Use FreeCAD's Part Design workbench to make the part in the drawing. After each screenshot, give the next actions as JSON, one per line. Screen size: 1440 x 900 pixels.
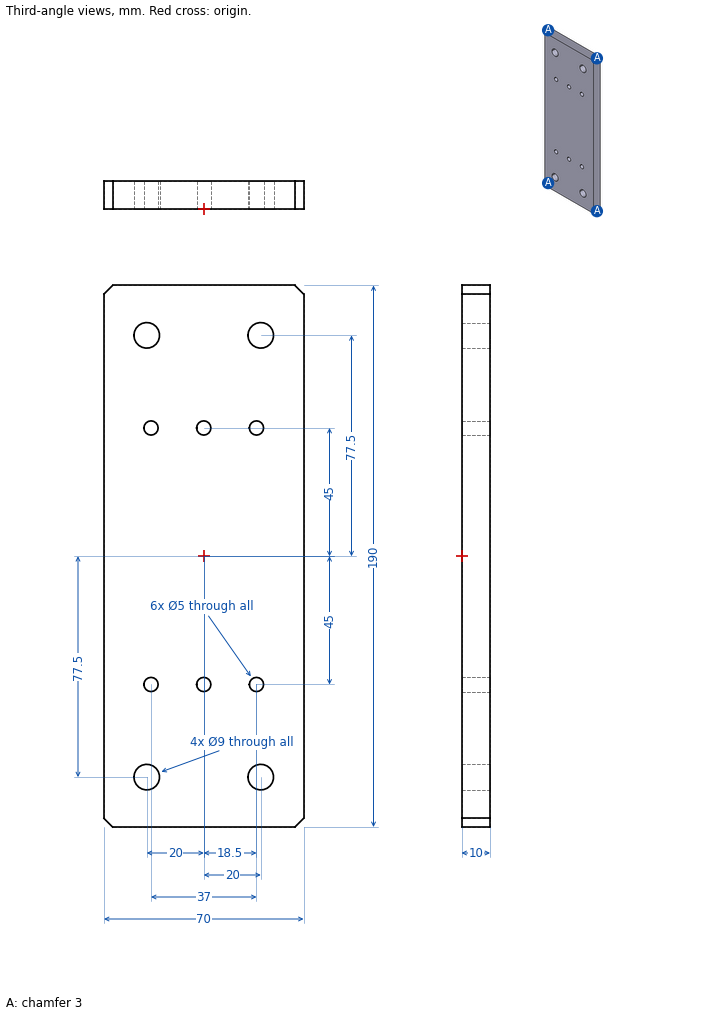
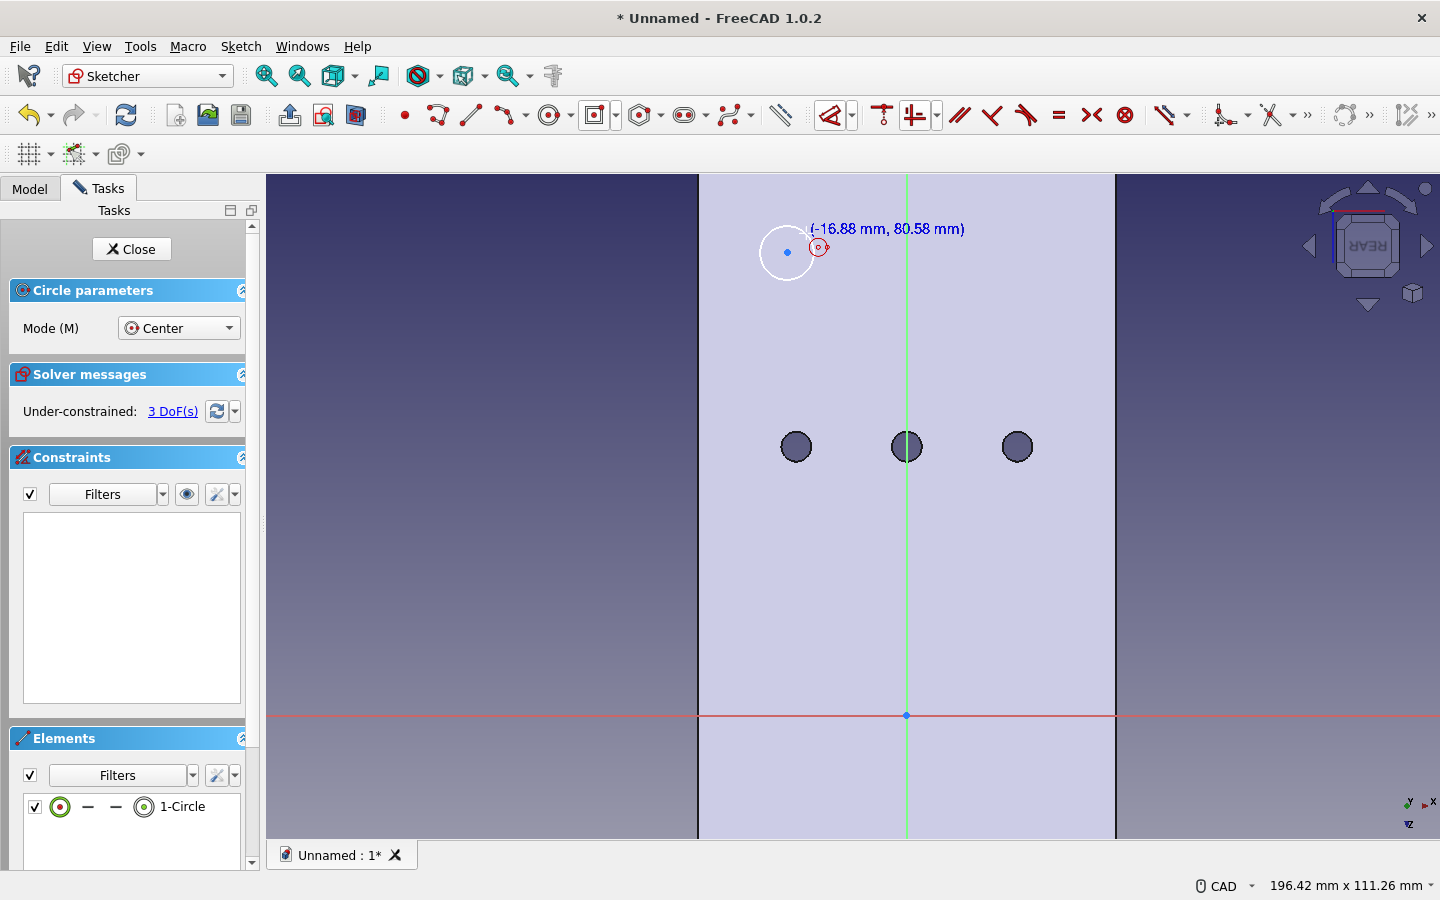
{"action": "left_click", "coordinate": [1026, 252]}
{"action": "left_click", "coordinate": [1045, 233]}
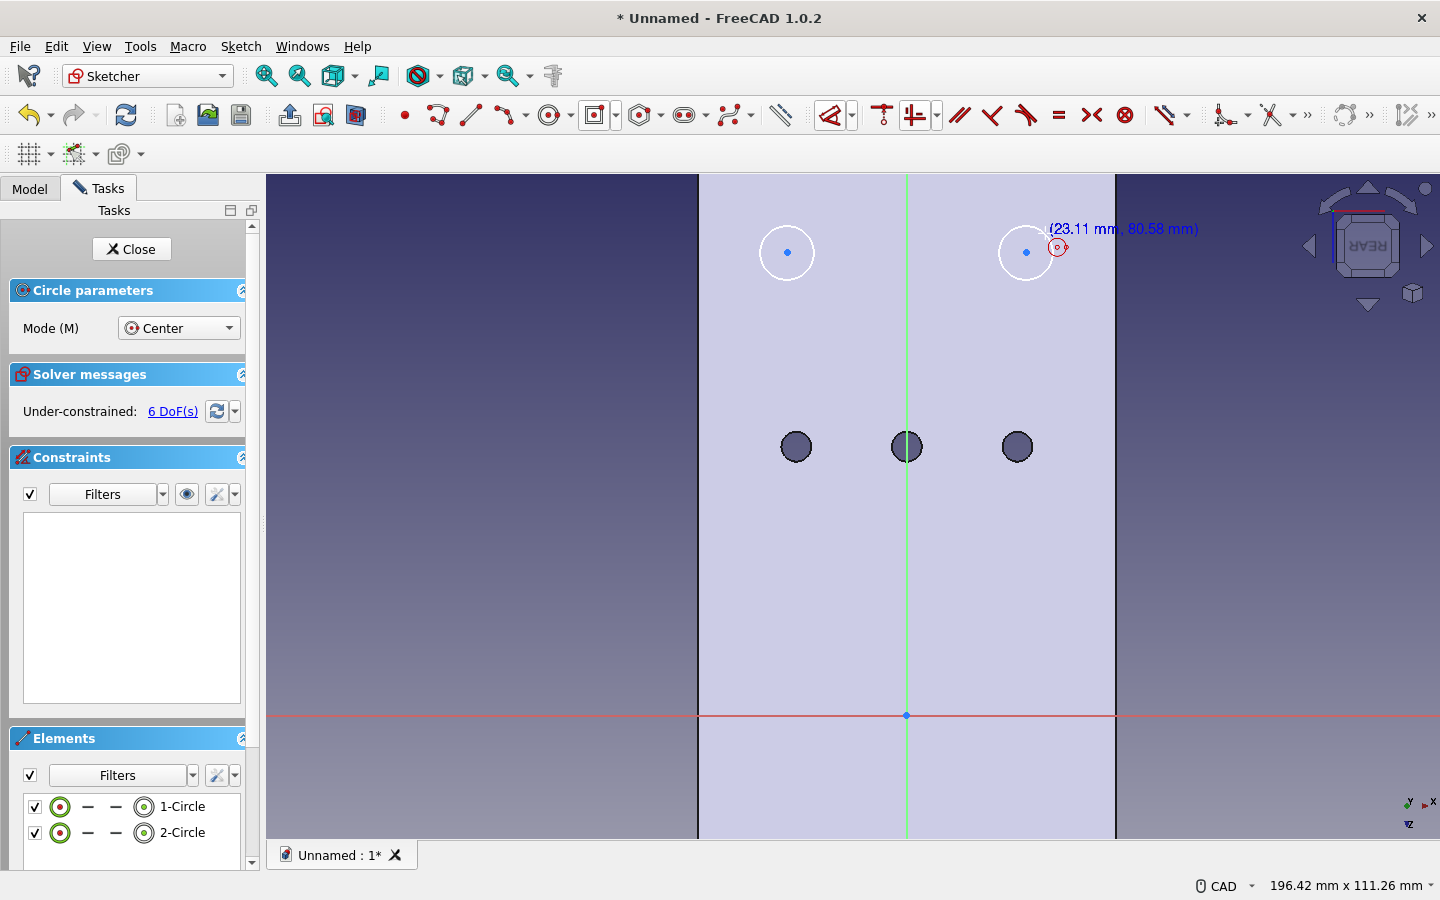
{"action": "scroll", "coordinate": [685, 336], "scroll_direction": "down", "scroll_amount": 4}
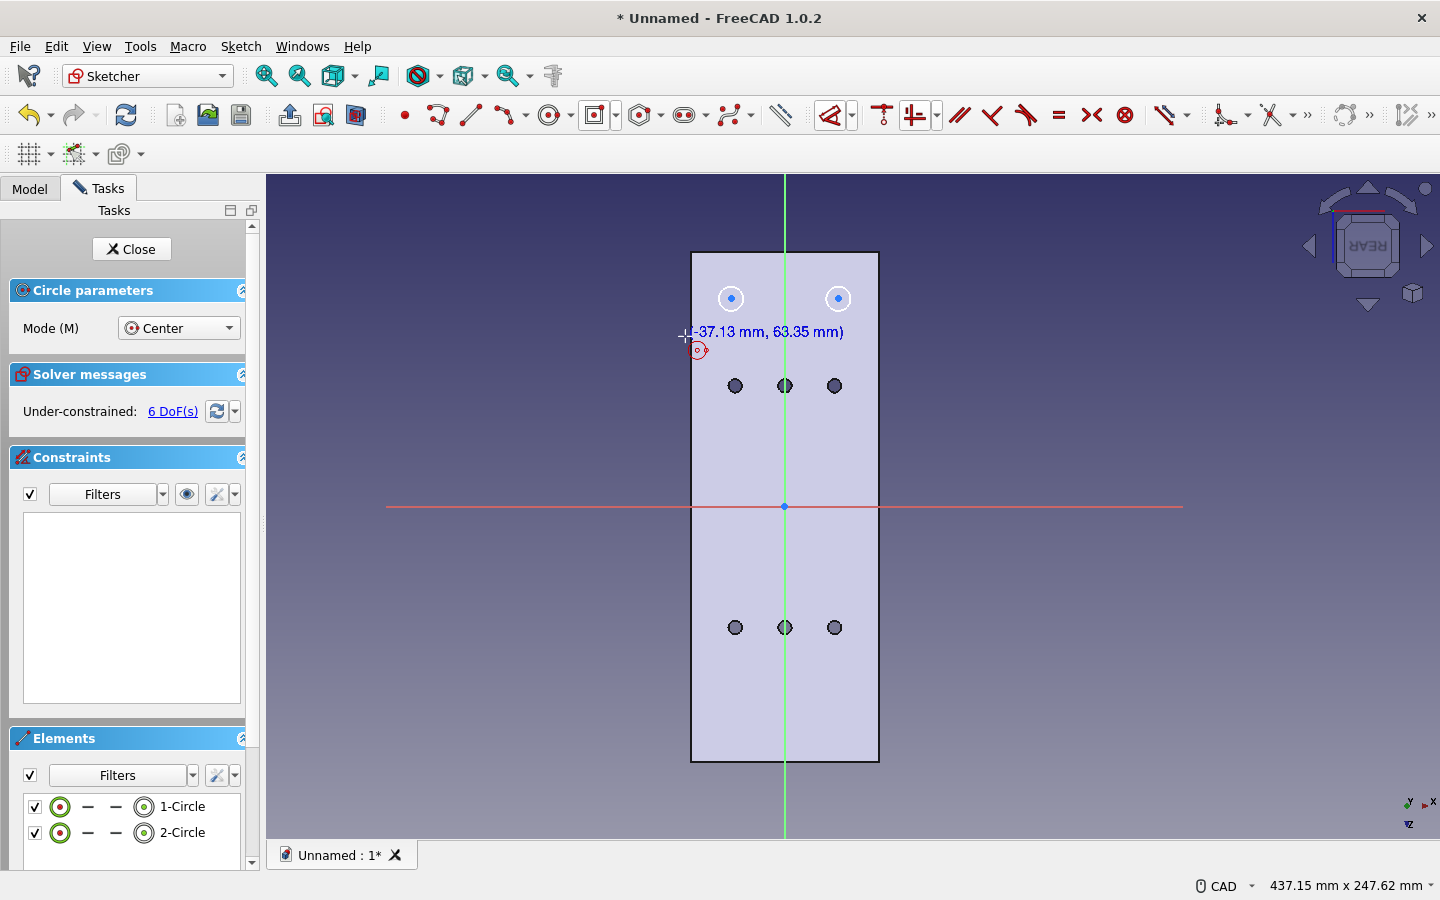
{"action": "scroll", "coordinate": [839, 715], "scroll_direction": "up", "scroll_amount": 4}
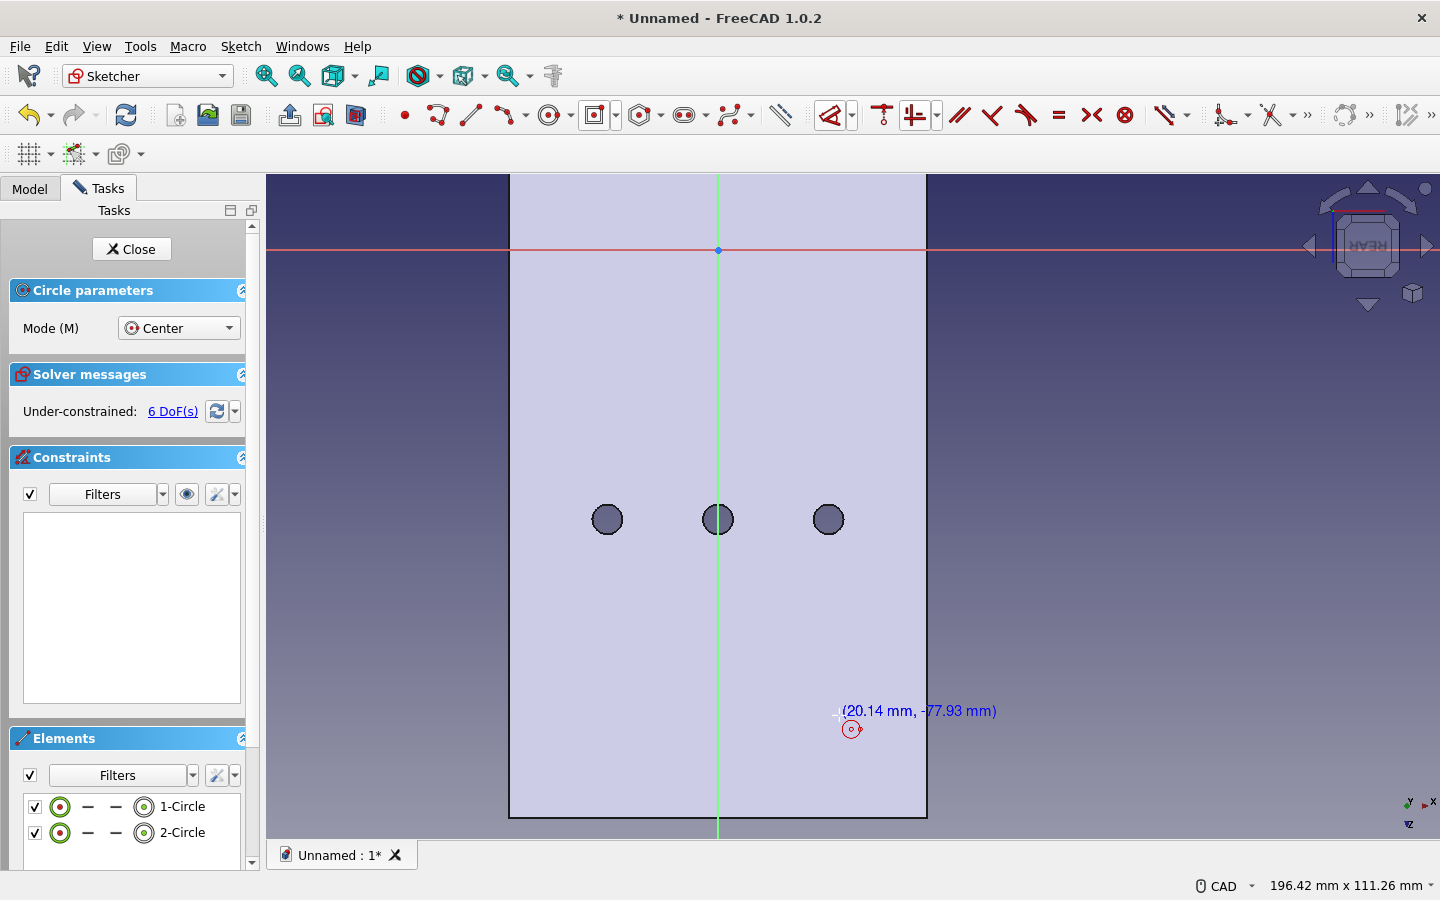
{"action": "left_click", "coordinate": [838, 714]}
{"action": "left_click", "coordinate": [857, 695]}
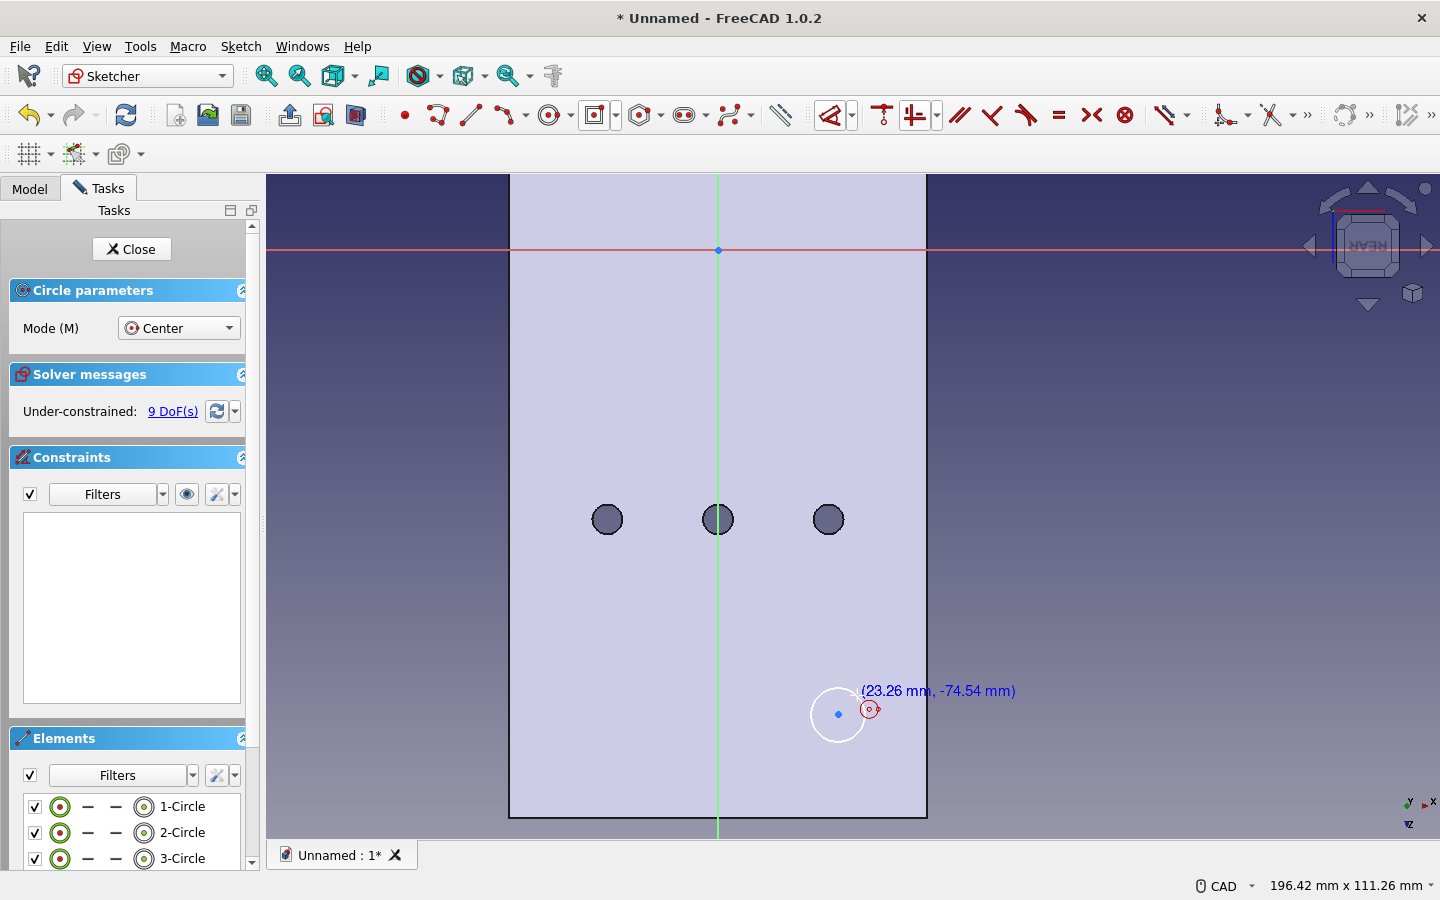
{"action": "left_click", "coordinate": [598, 714]}
{"action": "left_click", "coordinate": [617, 695]}
{"action": "key", "text": "Escape"}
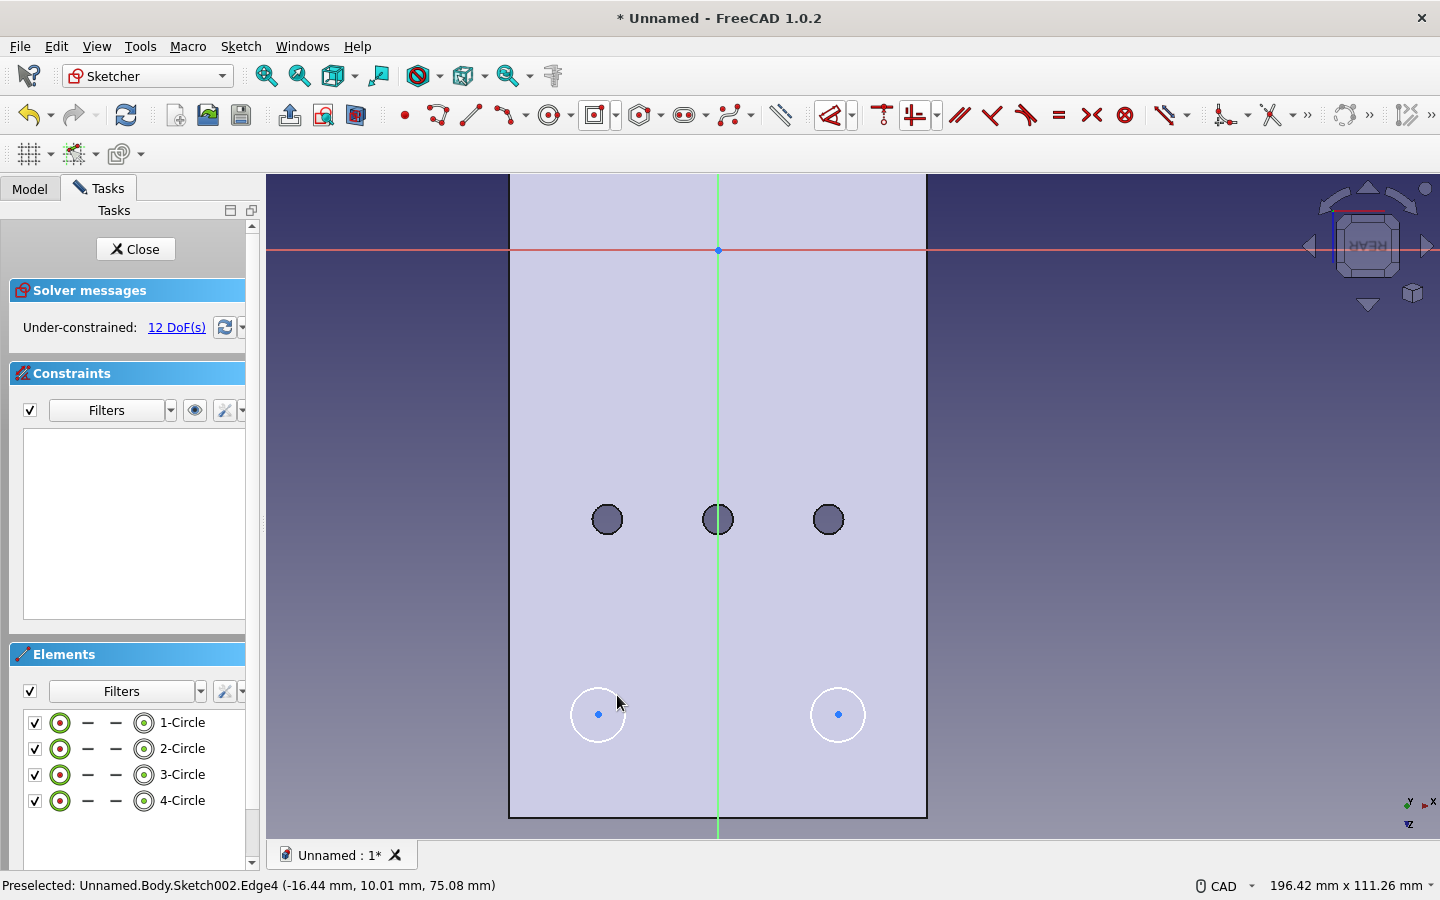
{"action": "scroll", "coordinate": [839, 715], "scroll_direction": "down", "scroll_amount": 4}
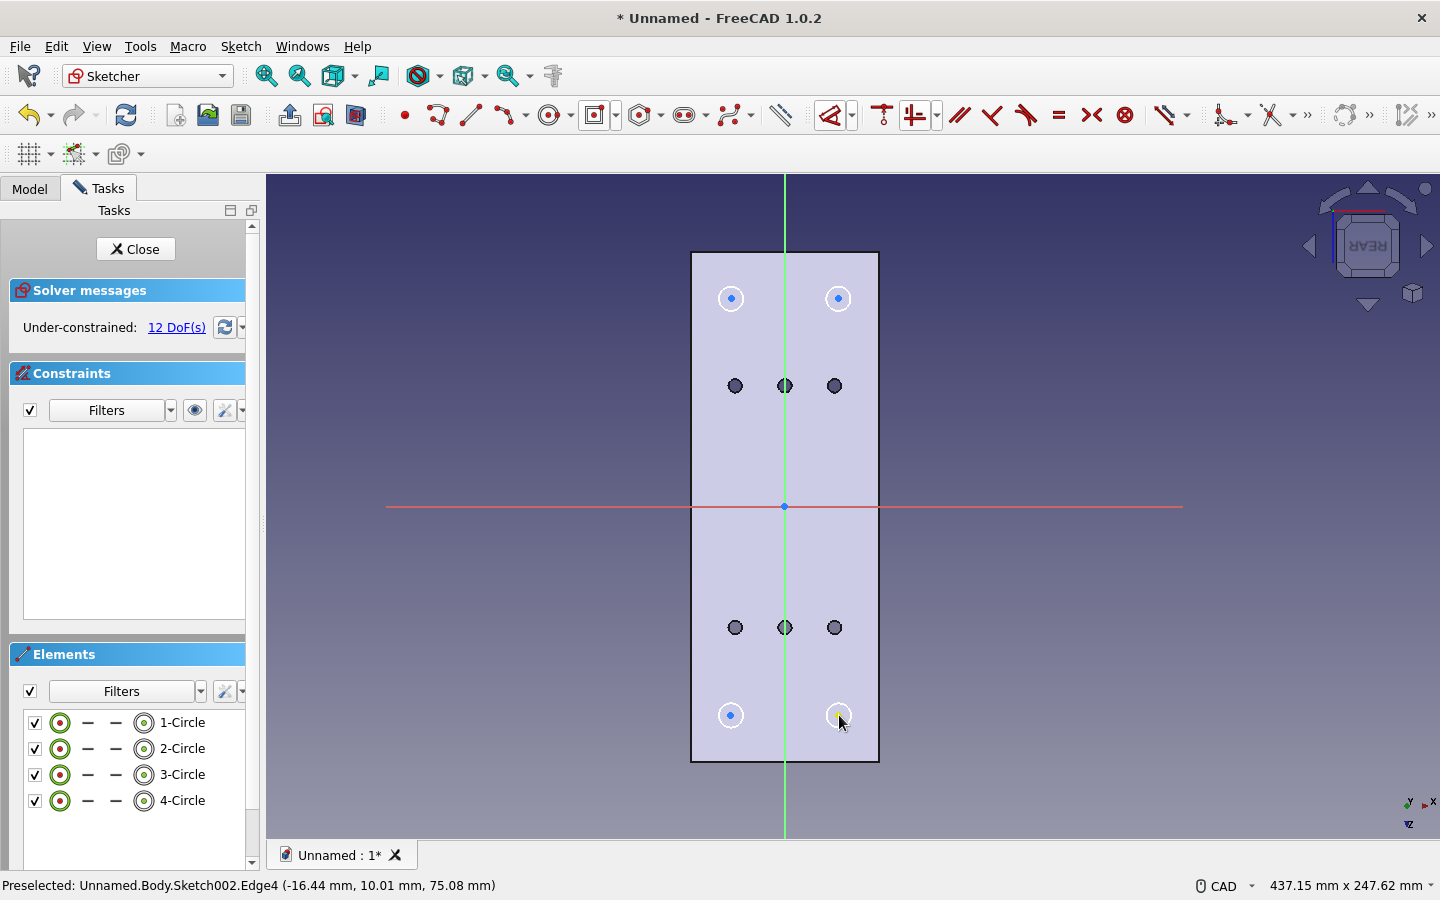
{"action": "left_click", "coordinate": [740, 290]}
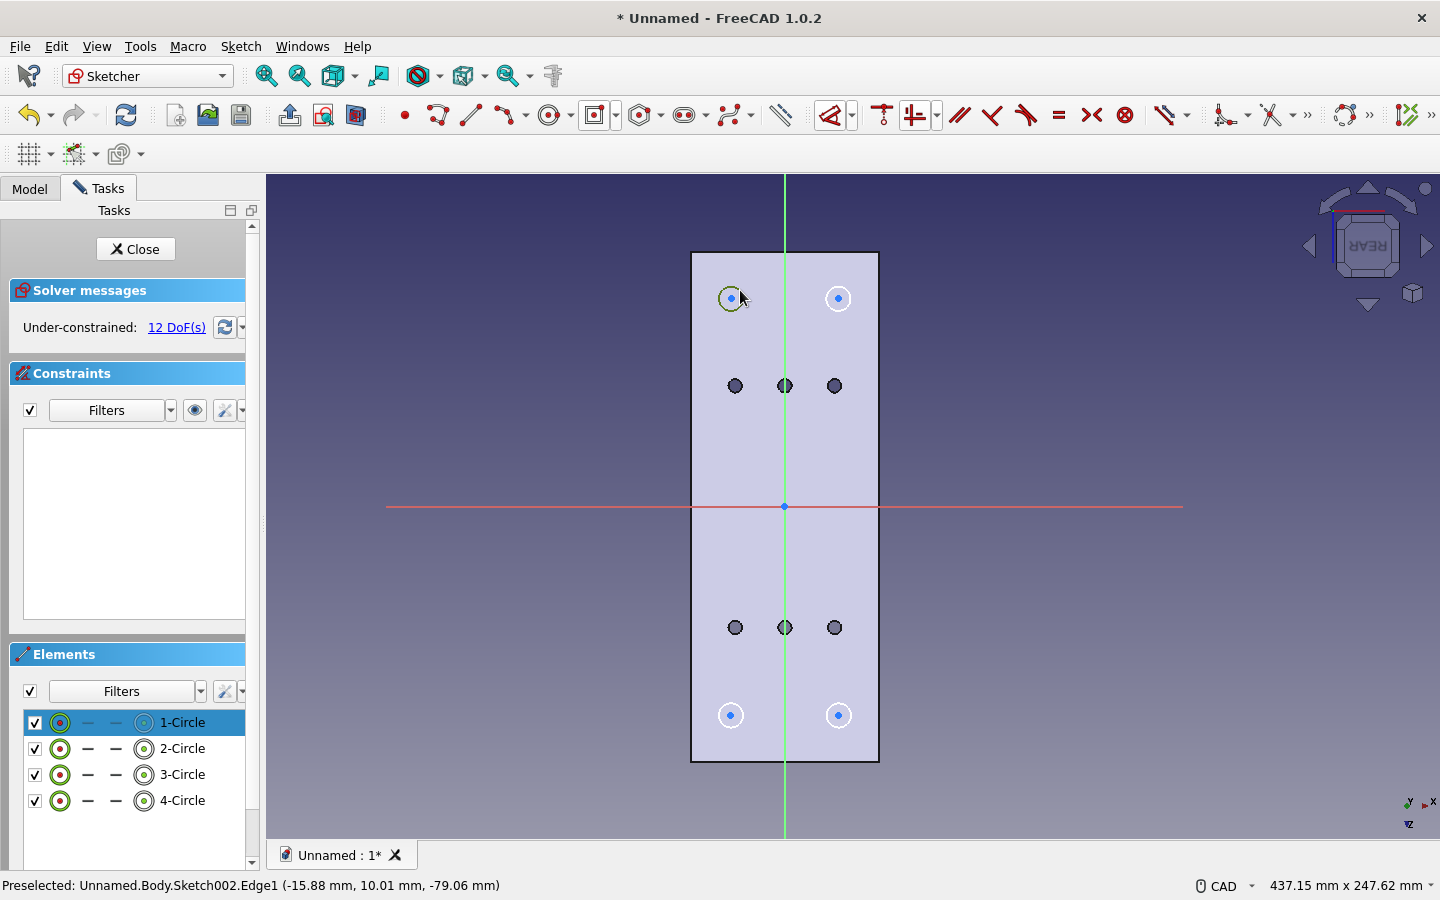
{"action": "left_click", "coordinate": [847, 290]}